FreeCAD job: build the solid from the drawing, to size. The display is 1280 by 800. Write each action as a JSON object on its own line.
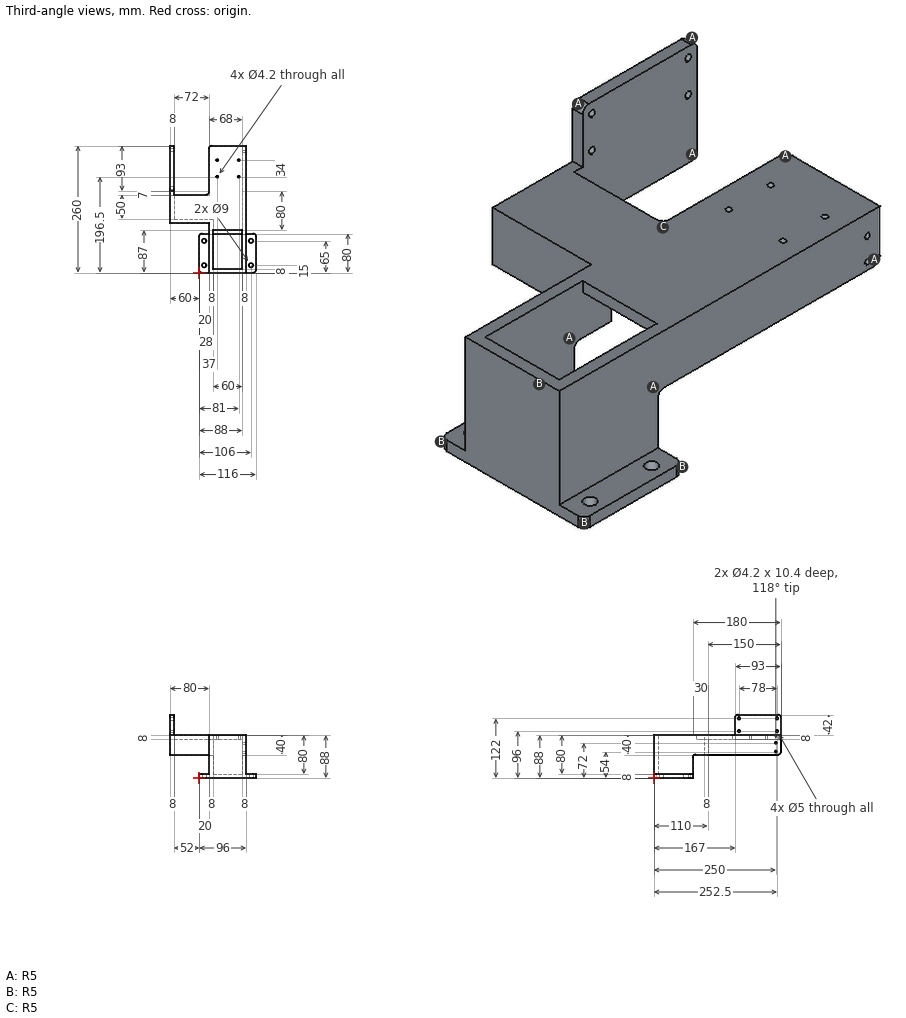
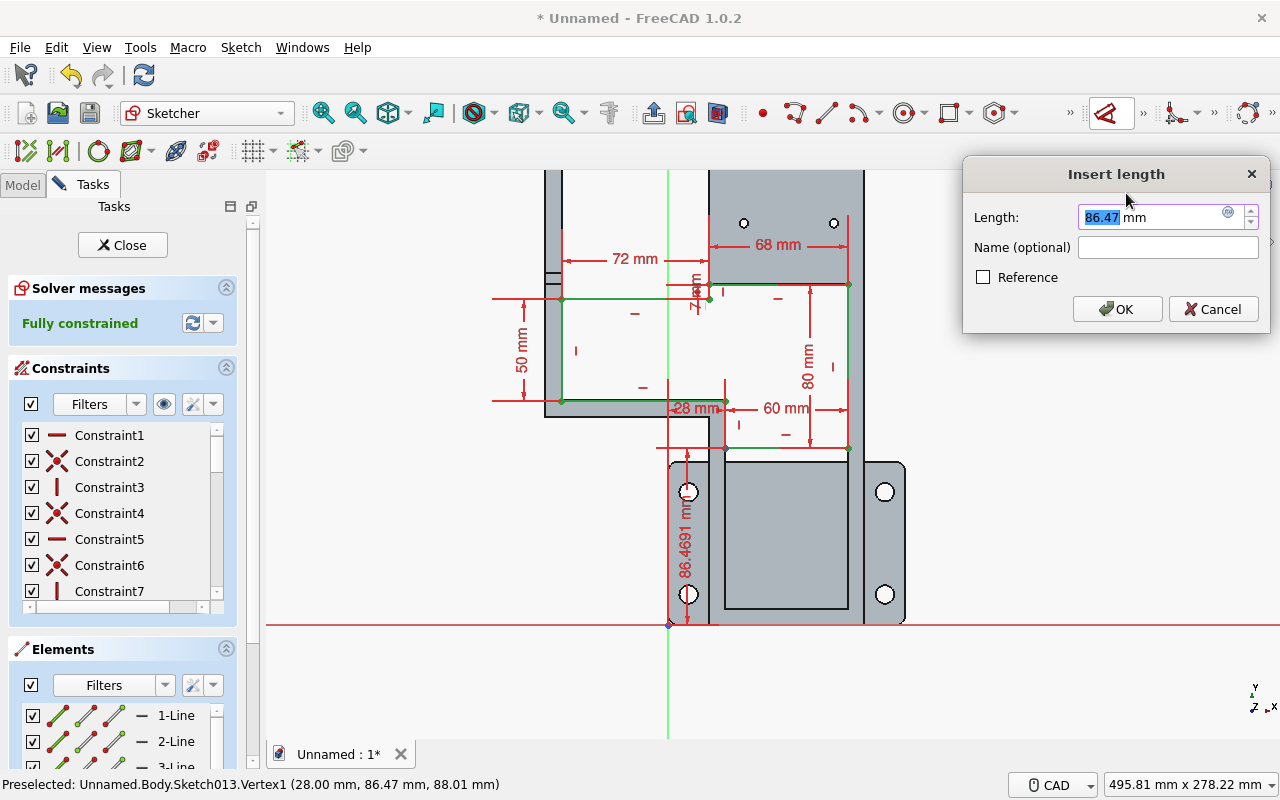
{"action": "type", "text": "87"}
{"action": "key", "text": "Return"}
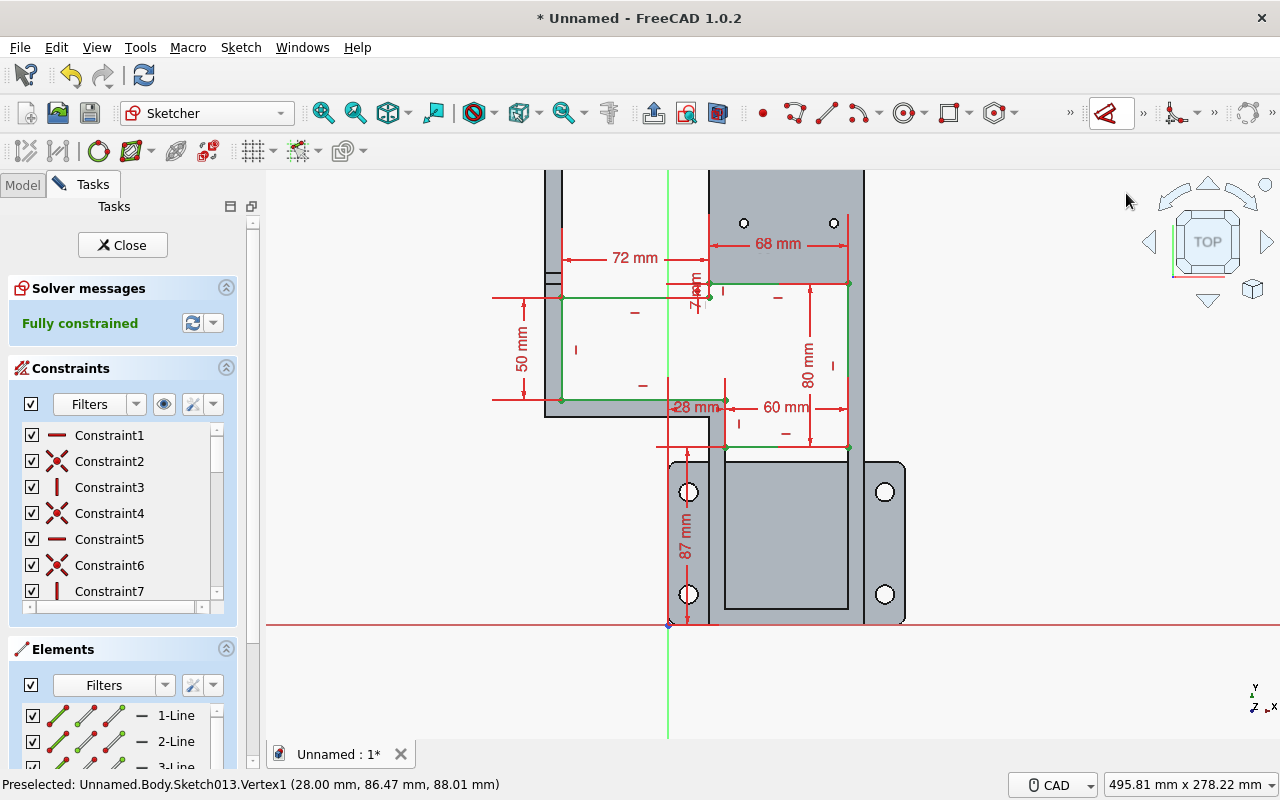
{"action": "left_click", "coordinate": [123, 245]}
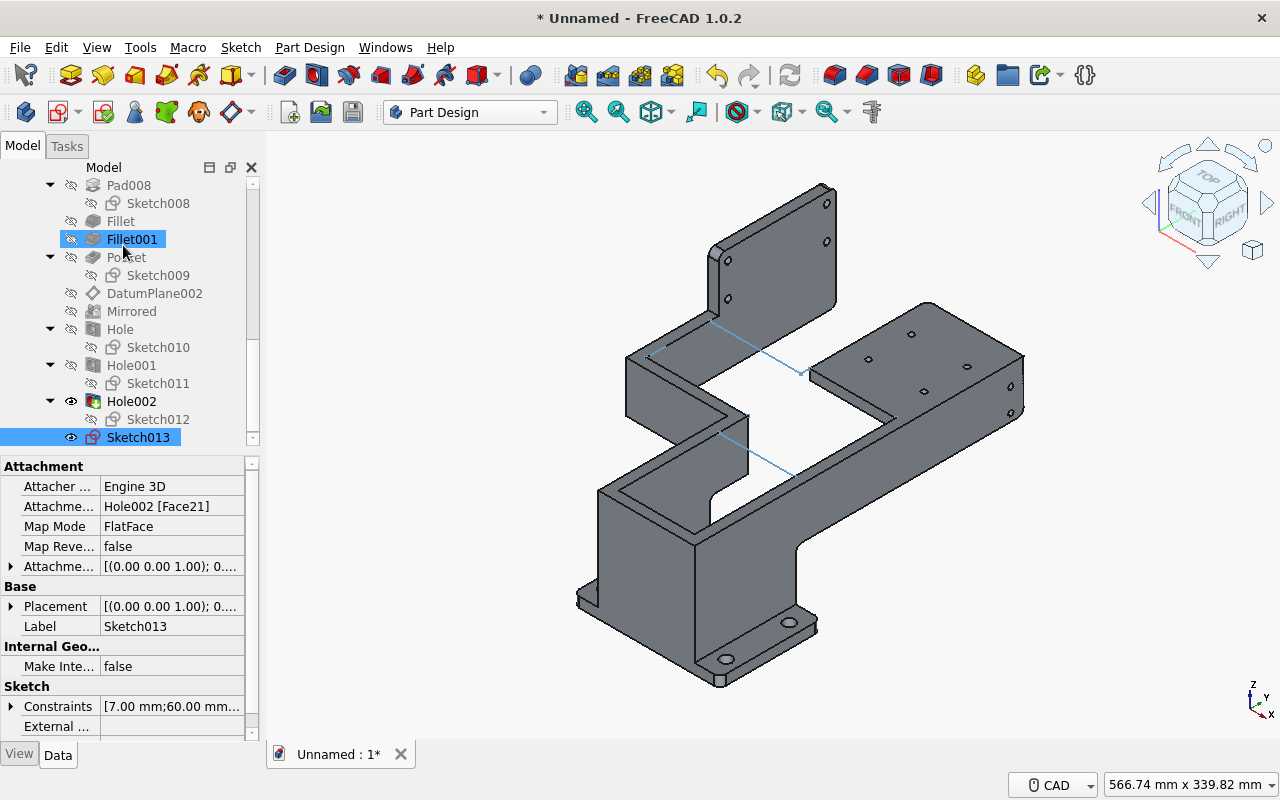
{"action": "left_click", "coordinate": [72, 76]}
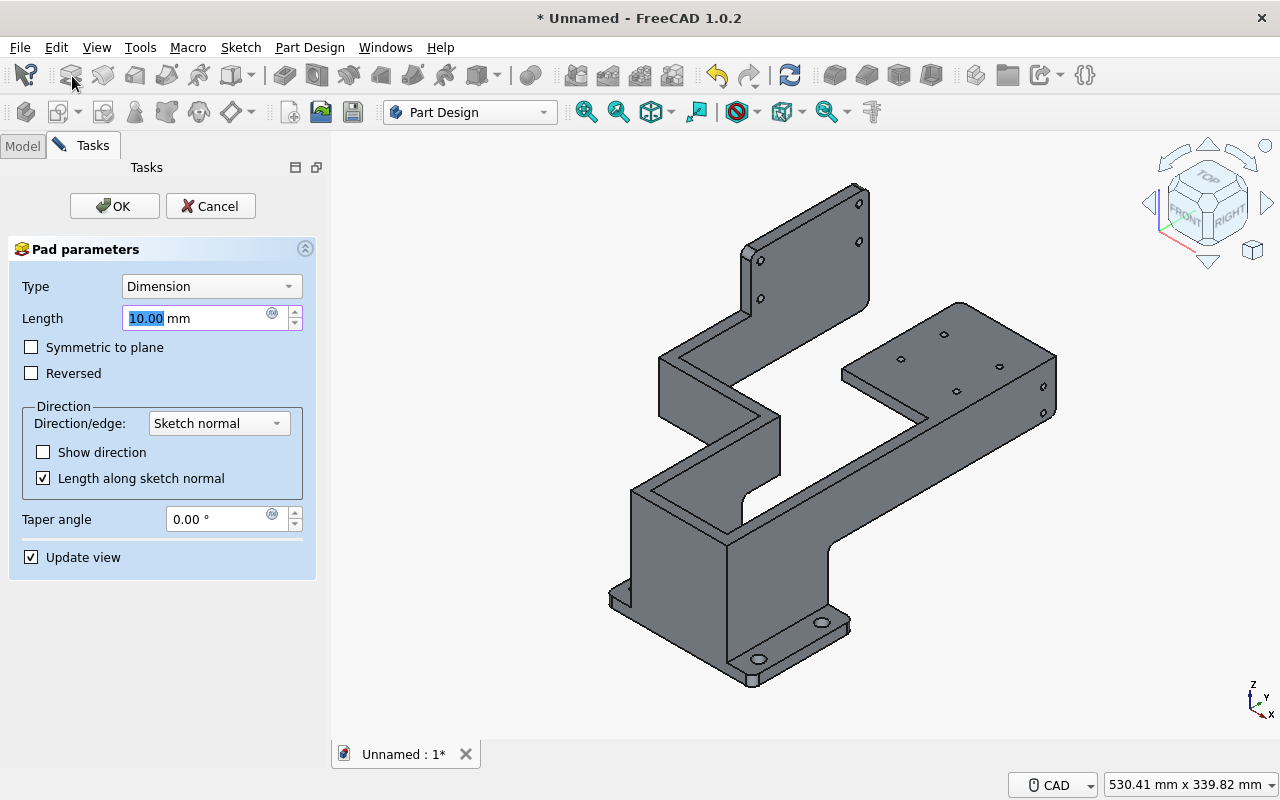
{"action": "type", "text": "8"}
{"action": "key", "text": "Tab"}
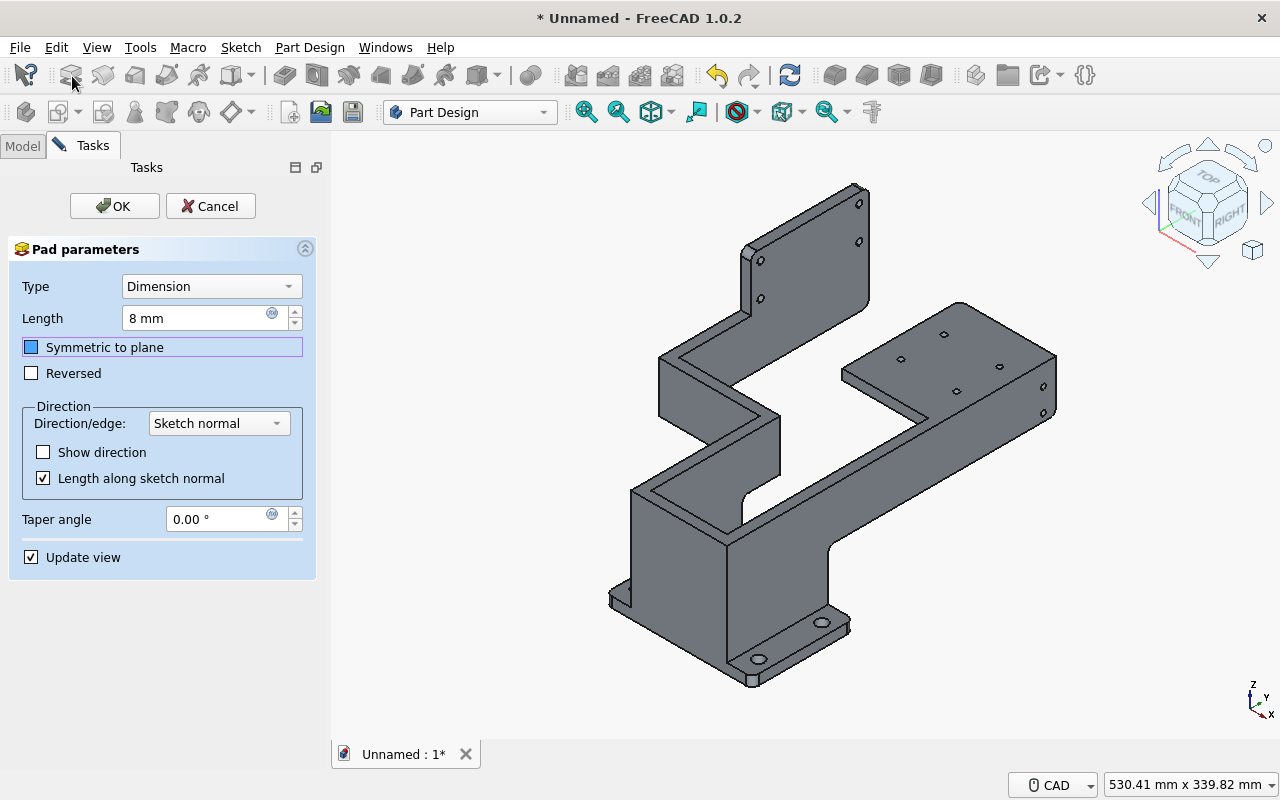
{"action": "left_click", "coordinate": [30, 373]}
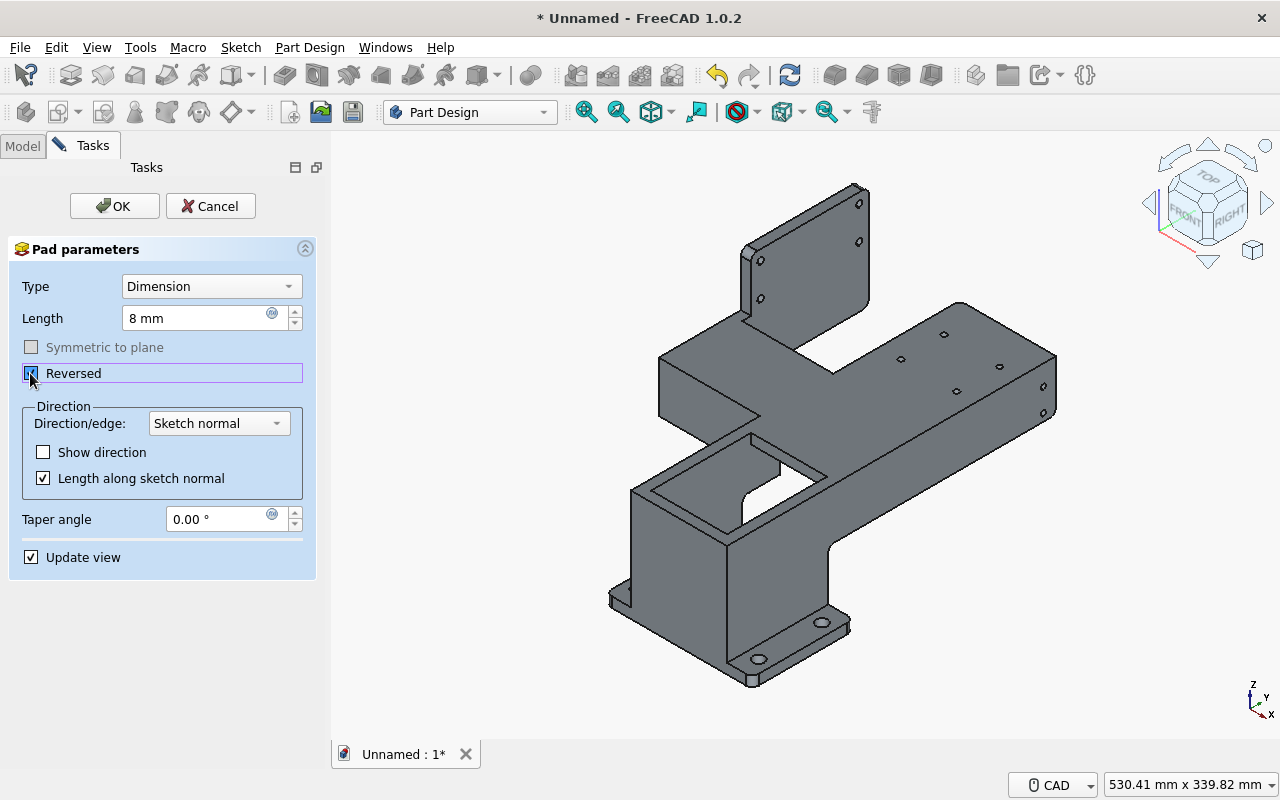
{"action": "left_click", "coordinate": [115, 206]}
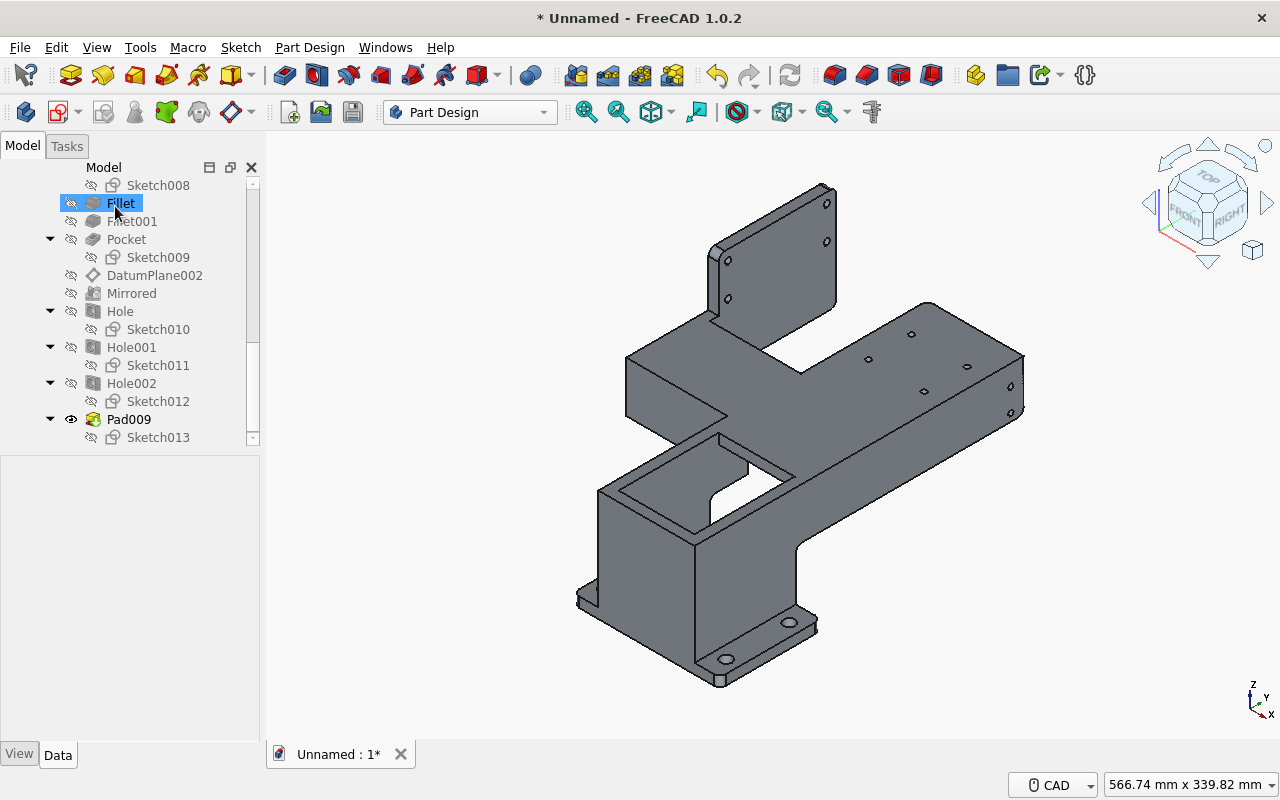
{"action": "scroll", "coordinate": [801, 378], "scroll_direction": "up", "scroll_amount": 6}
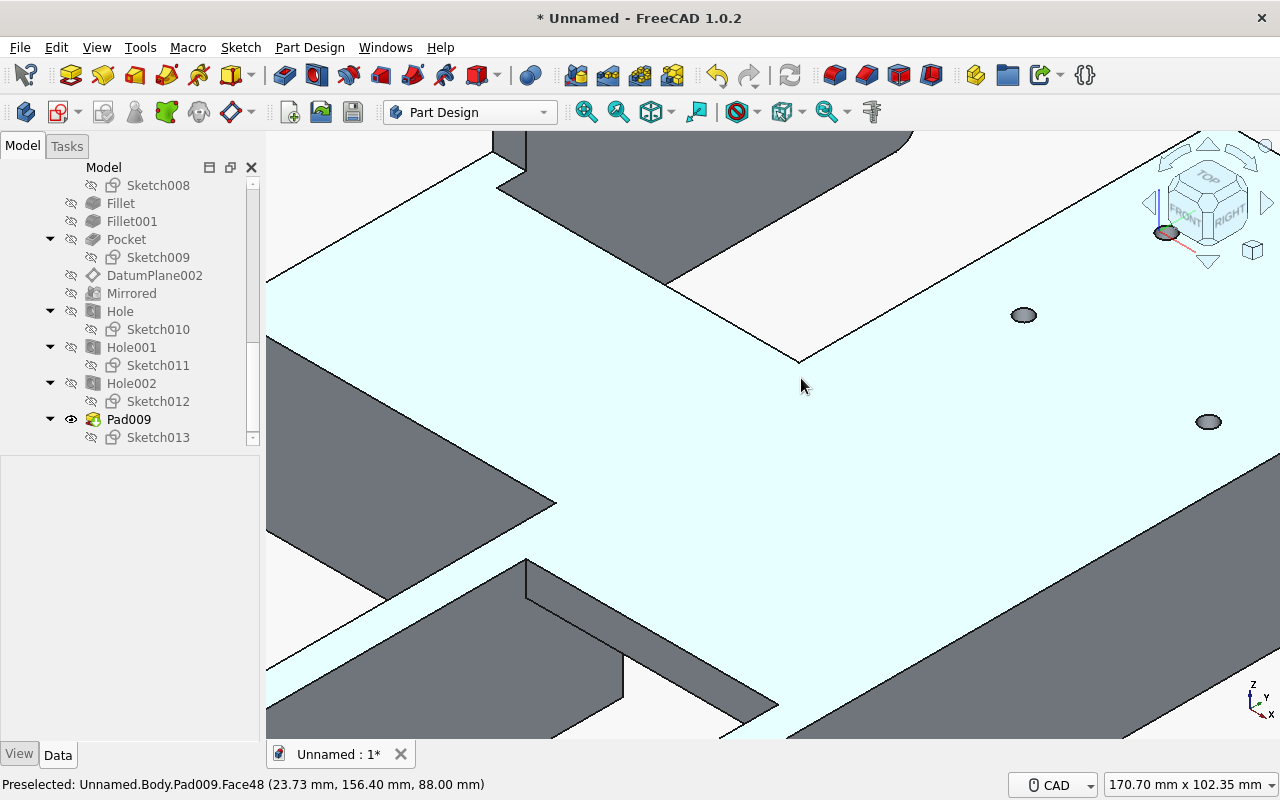
{"action": "left_click", "coordinate": [588, 112]}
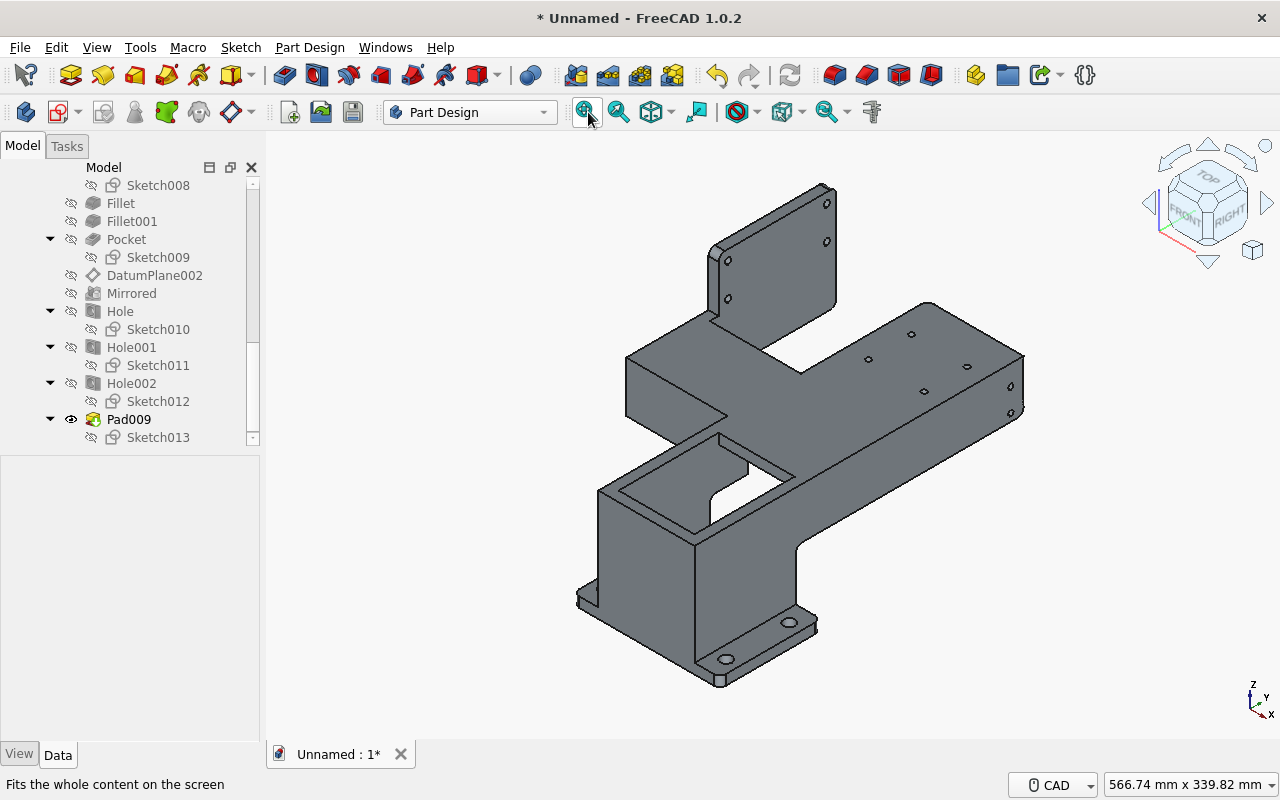
{"action": "key", "text": "2"}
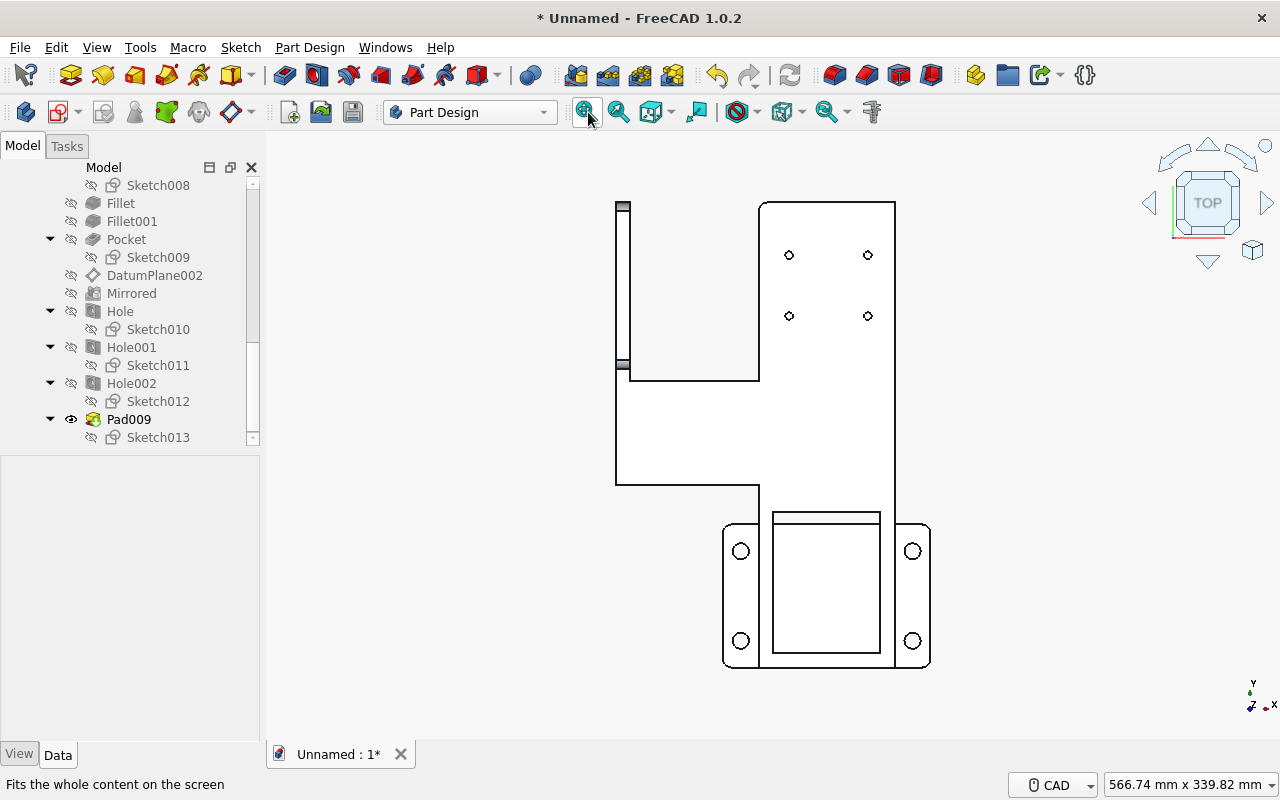
{"action": "scroll", "coordinate": [759, 380], "scroll_direction": "up", "scroll_amount": 6}